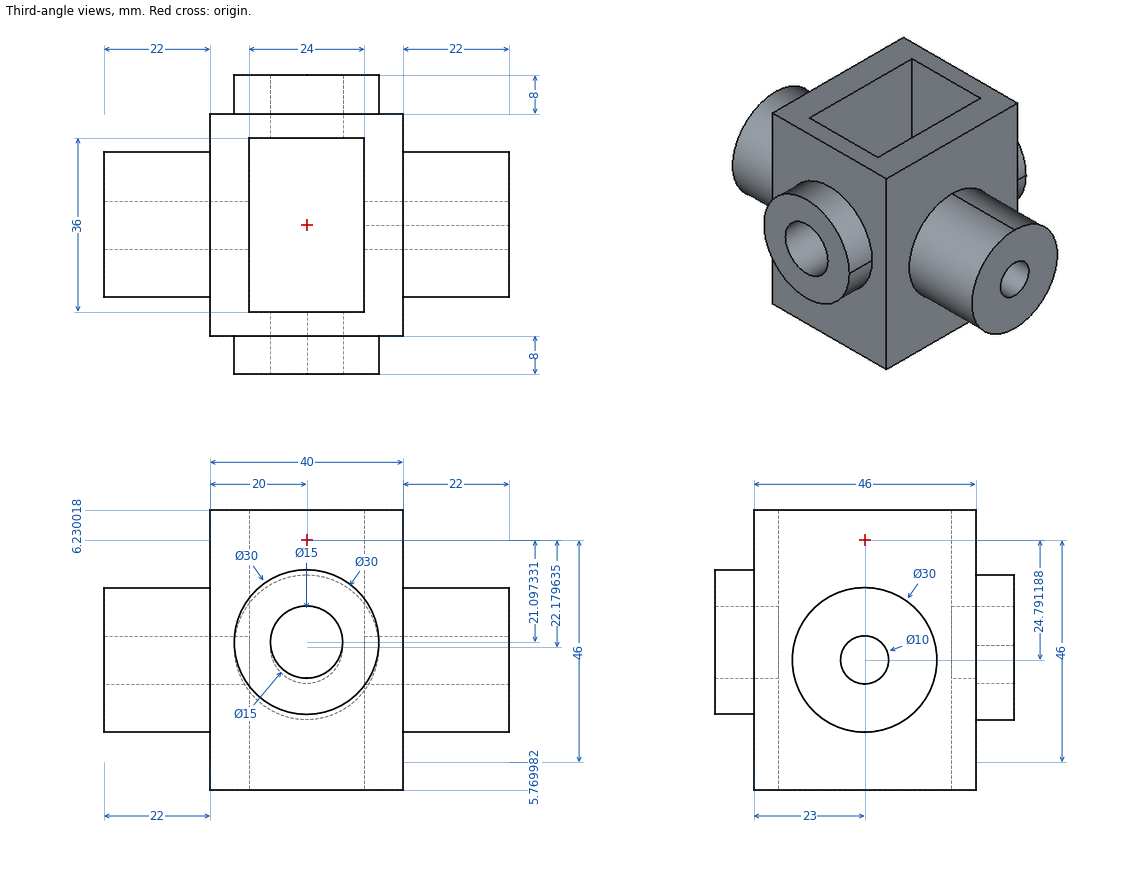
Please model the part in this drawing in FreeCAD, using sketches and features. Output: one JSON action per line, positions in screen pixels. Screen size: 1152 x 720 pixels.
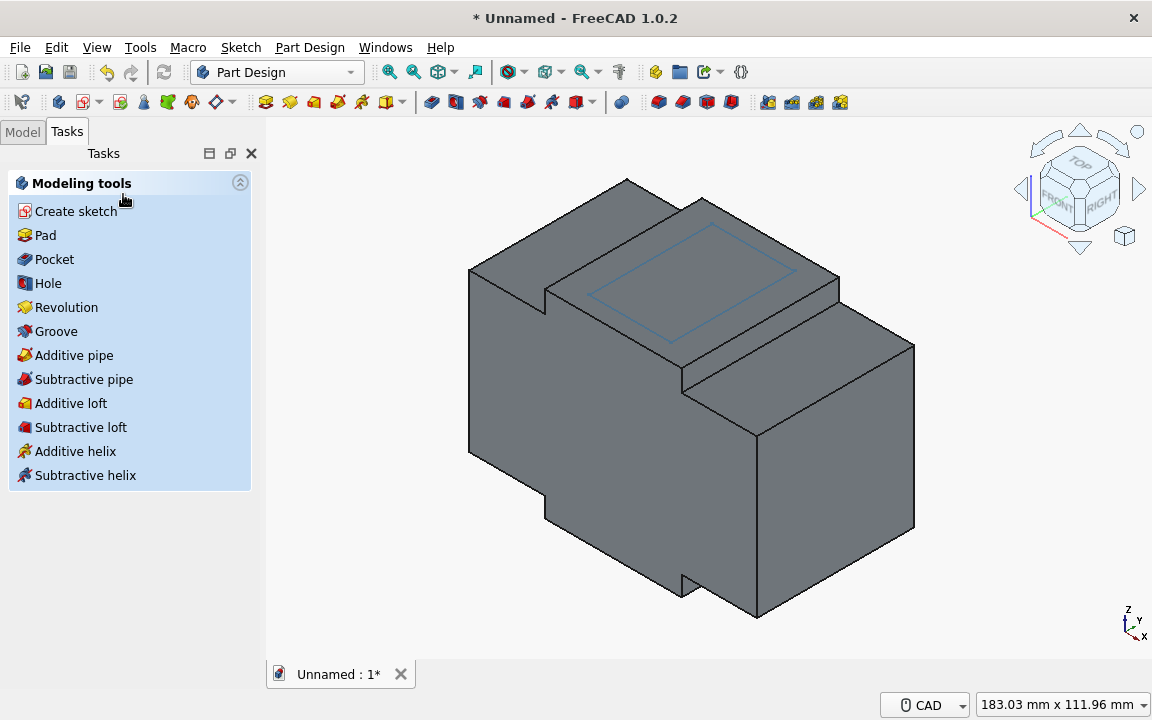
{"action": "left_click", "coordinate": [432, 102]}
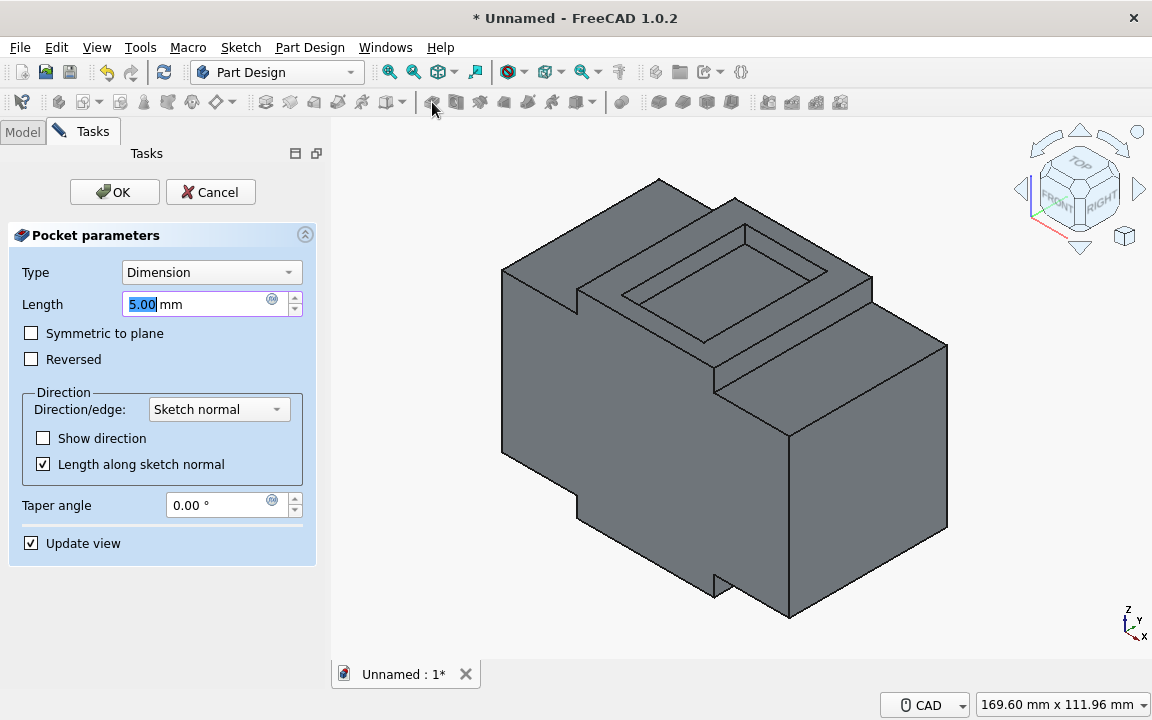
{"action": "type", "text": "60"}
{"action": "key", "text": "Tab"}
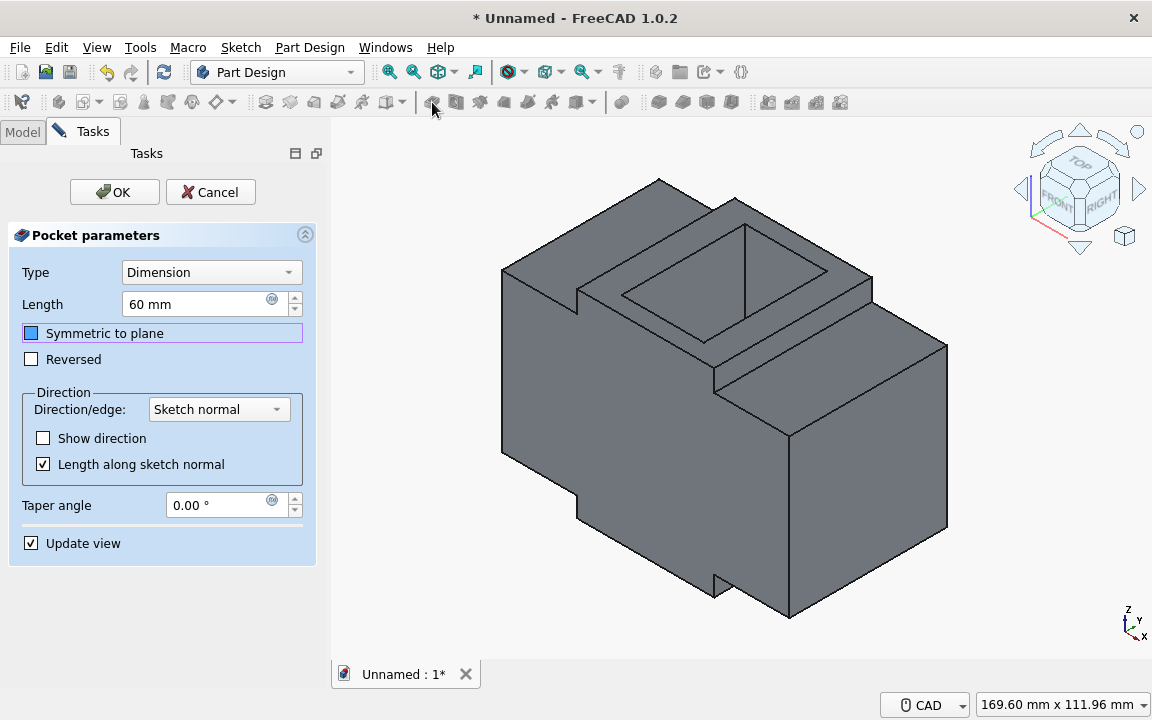
{"action": "left_click", "coordinate": [115, 192]}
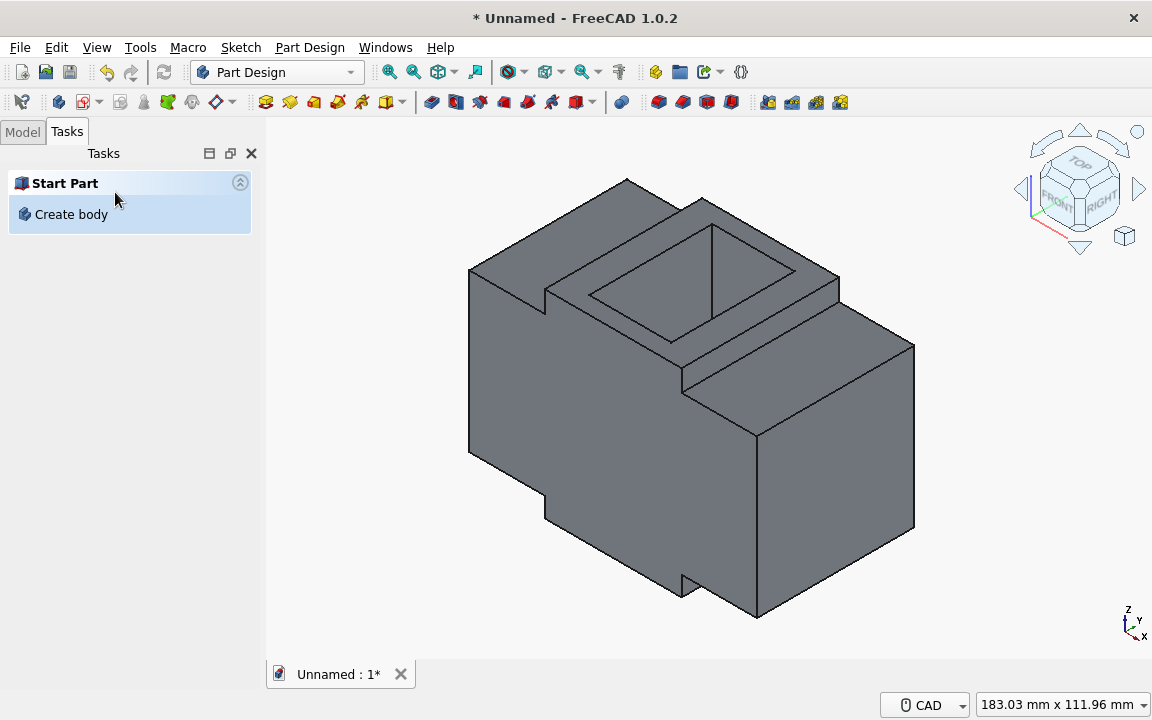
{"action": "left_click", "coordinate": [836, 481]}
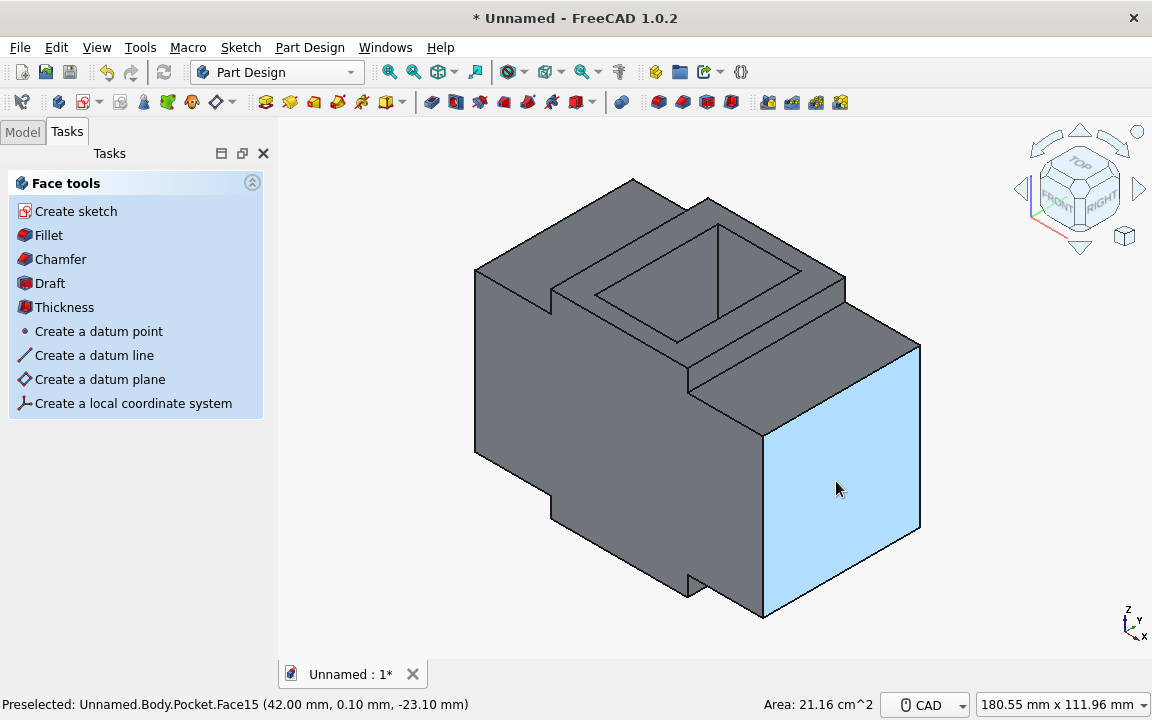
{"action": "left_click", "coordinate": [84, 102]}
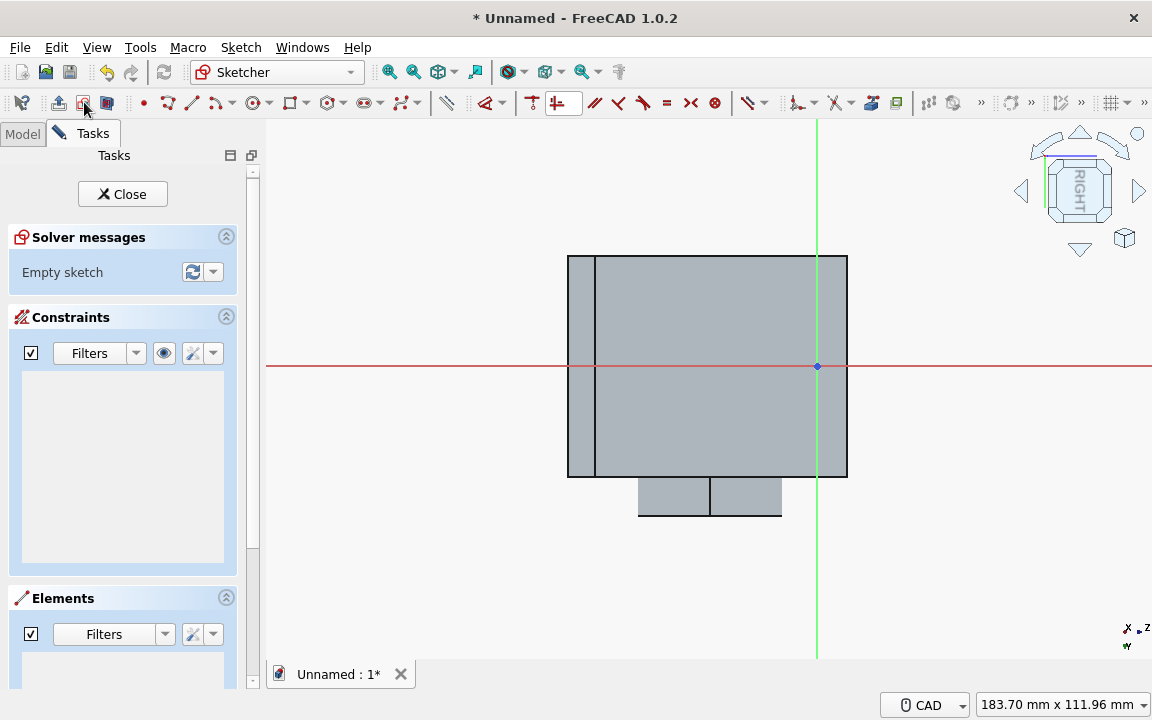
{"action": "scroll", "coordinate": [707, 363], "scroll_direction": "up", "scroll_amount": 10}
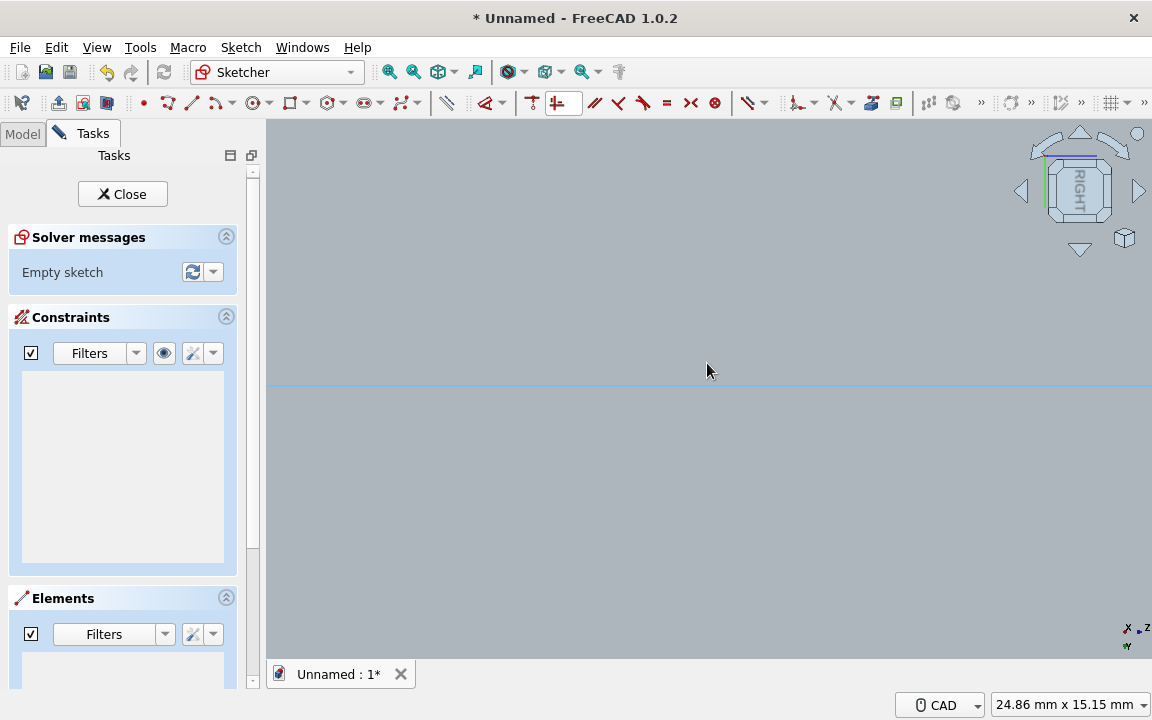
{"action": "left_click", "coordinate": [254, 104]}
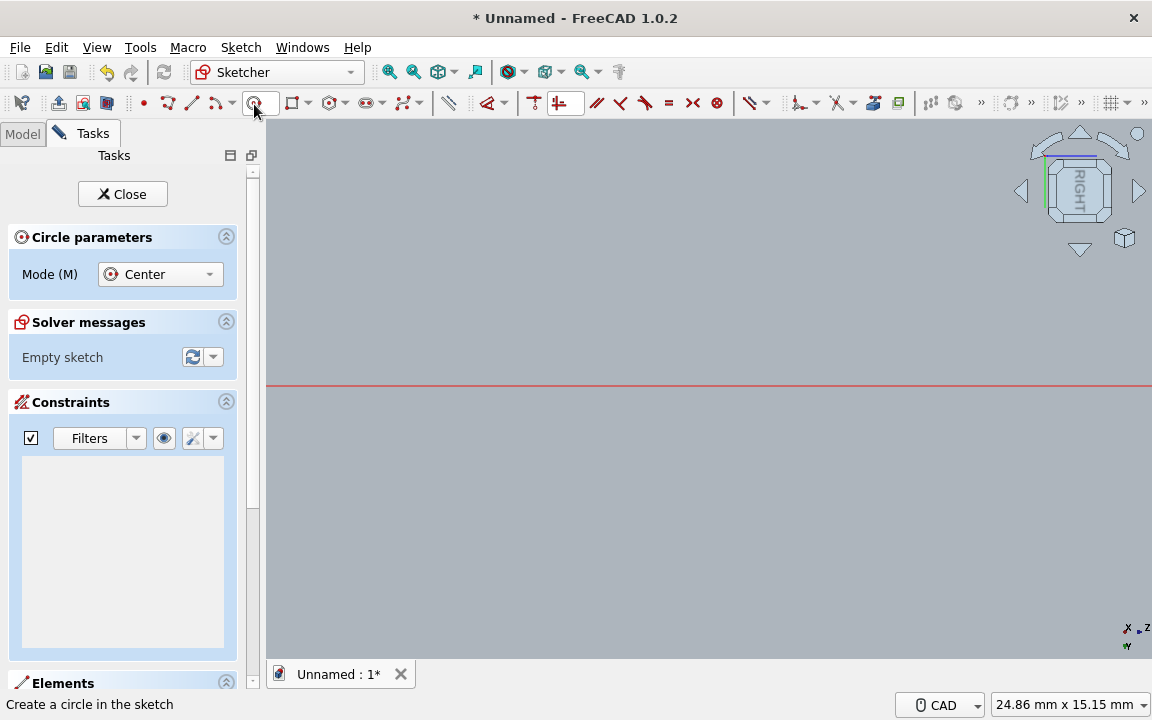
{"action": "left_click", "coordinate": [635, 386]}
{"action": "left_click", "coordinate": [761, 260]}
{"action": "key", "text": "Escape"}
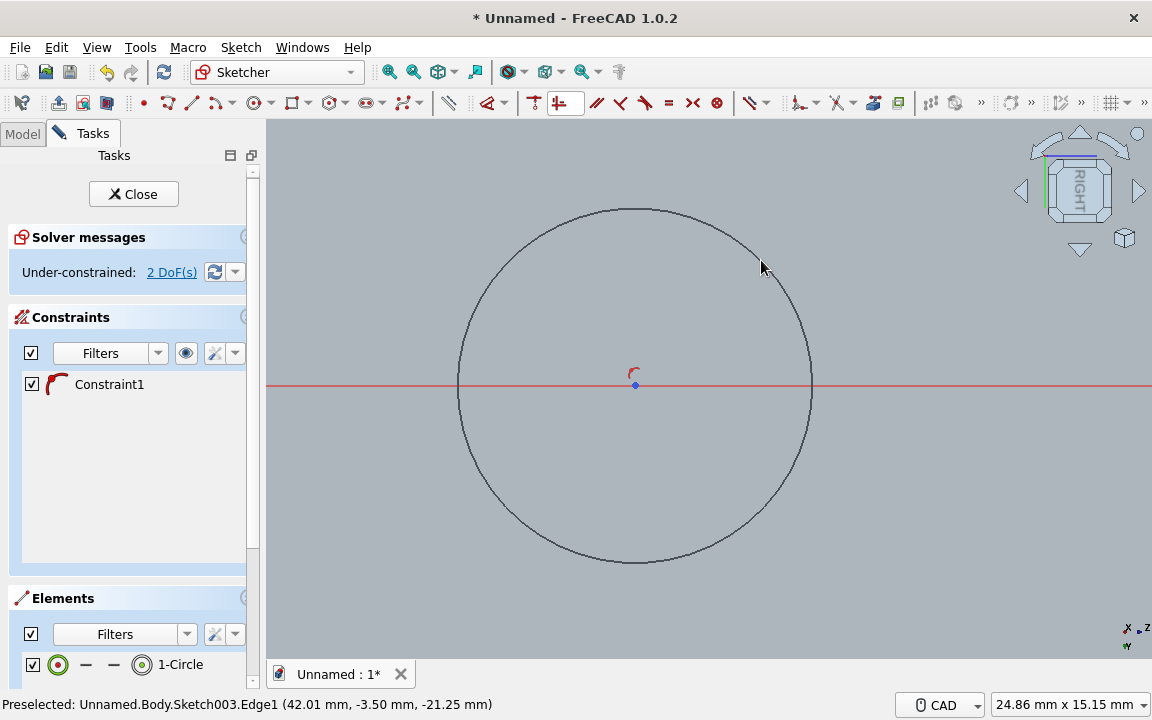
{"action": "left_click", "coordinate": [488, 104]}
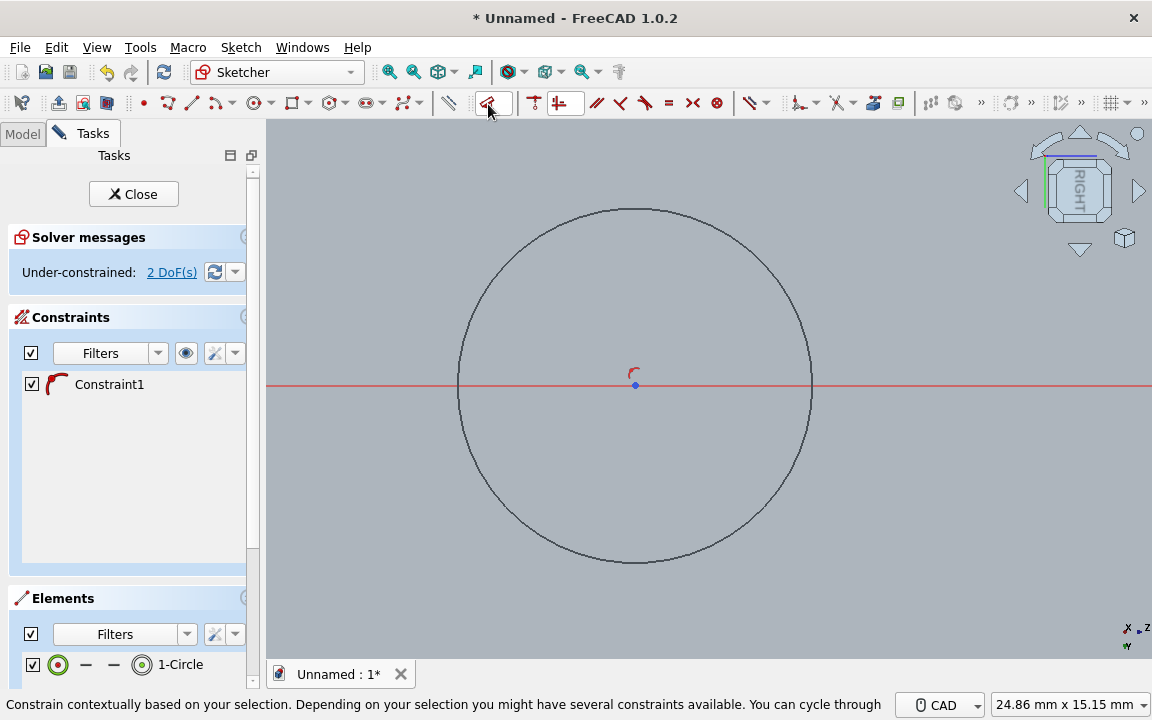
{"action": "left_click", "coordinate": [760, 260]}
{"action": "left_click", "coordinate": [783, 237]}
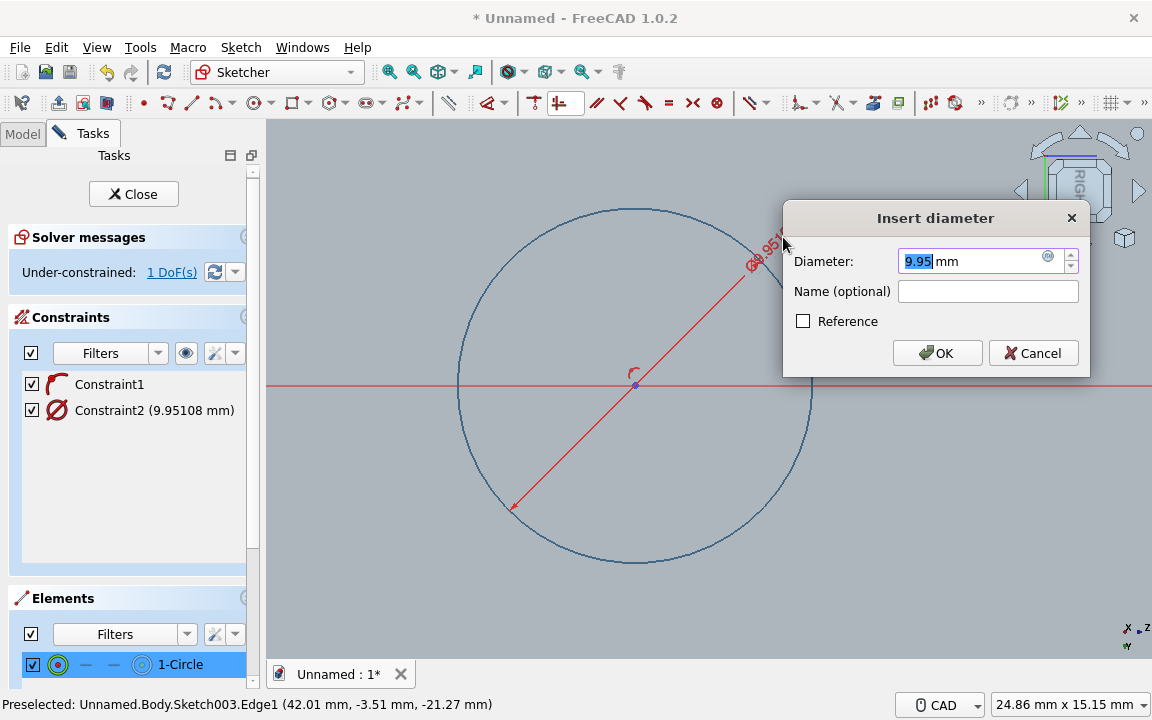
{"action": "type", "text": "10"}
{"action": "key", "text": "Return"}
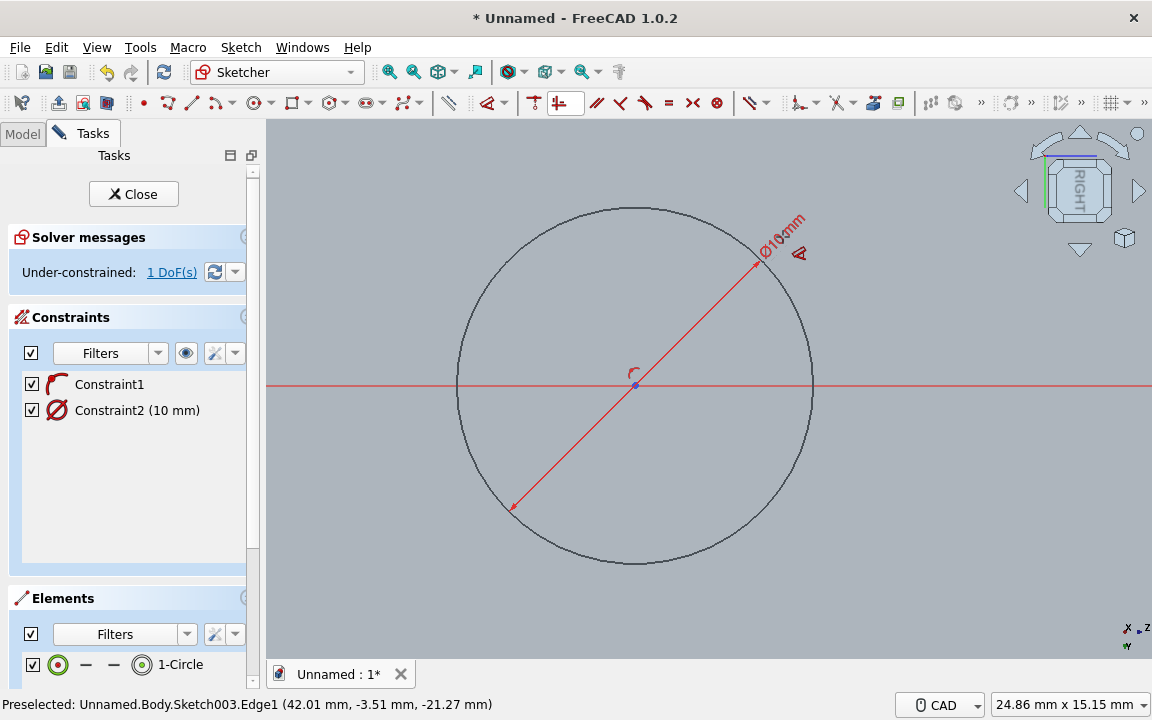
{"action": "left_click", "coordinate": [635, 386]}
{"action": "left_click", "coordinate": [730, 420]}